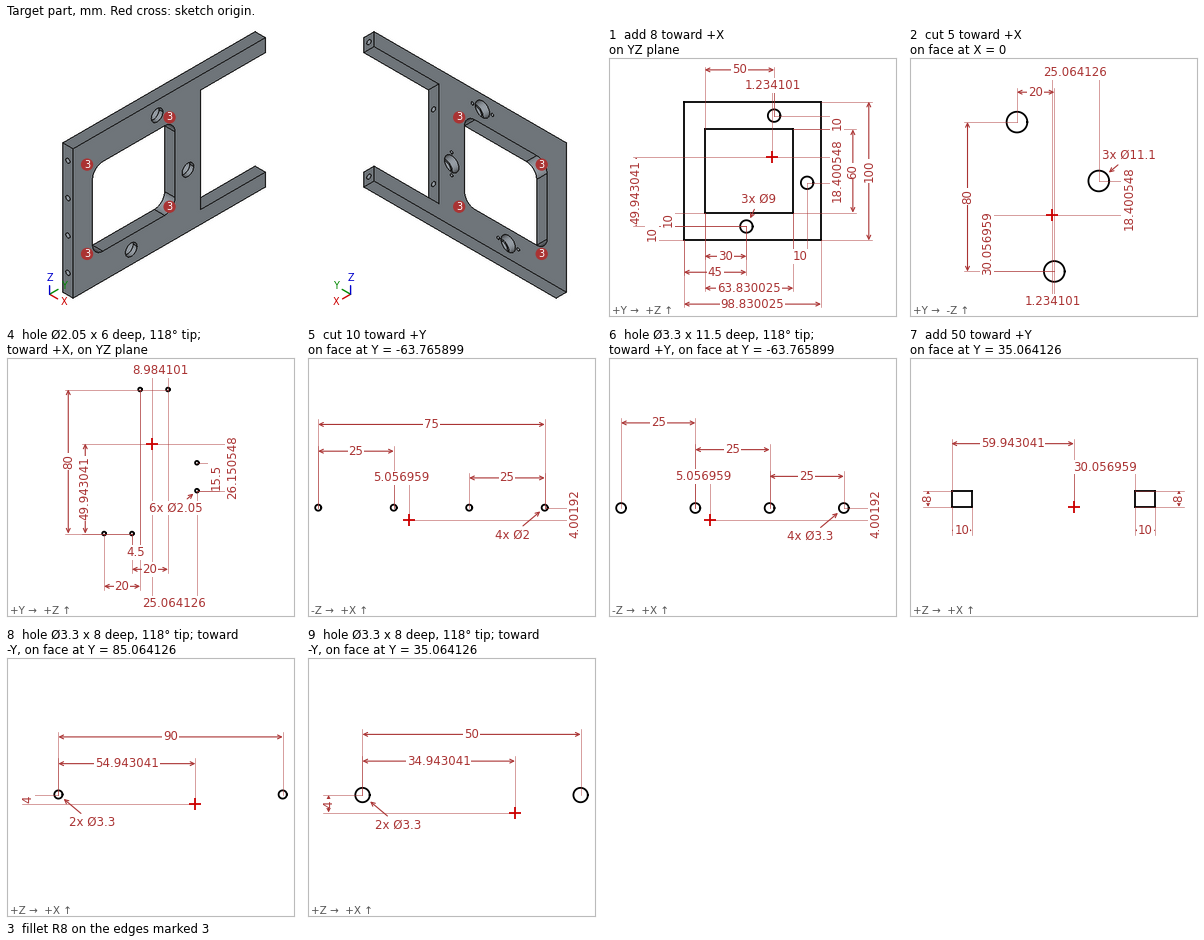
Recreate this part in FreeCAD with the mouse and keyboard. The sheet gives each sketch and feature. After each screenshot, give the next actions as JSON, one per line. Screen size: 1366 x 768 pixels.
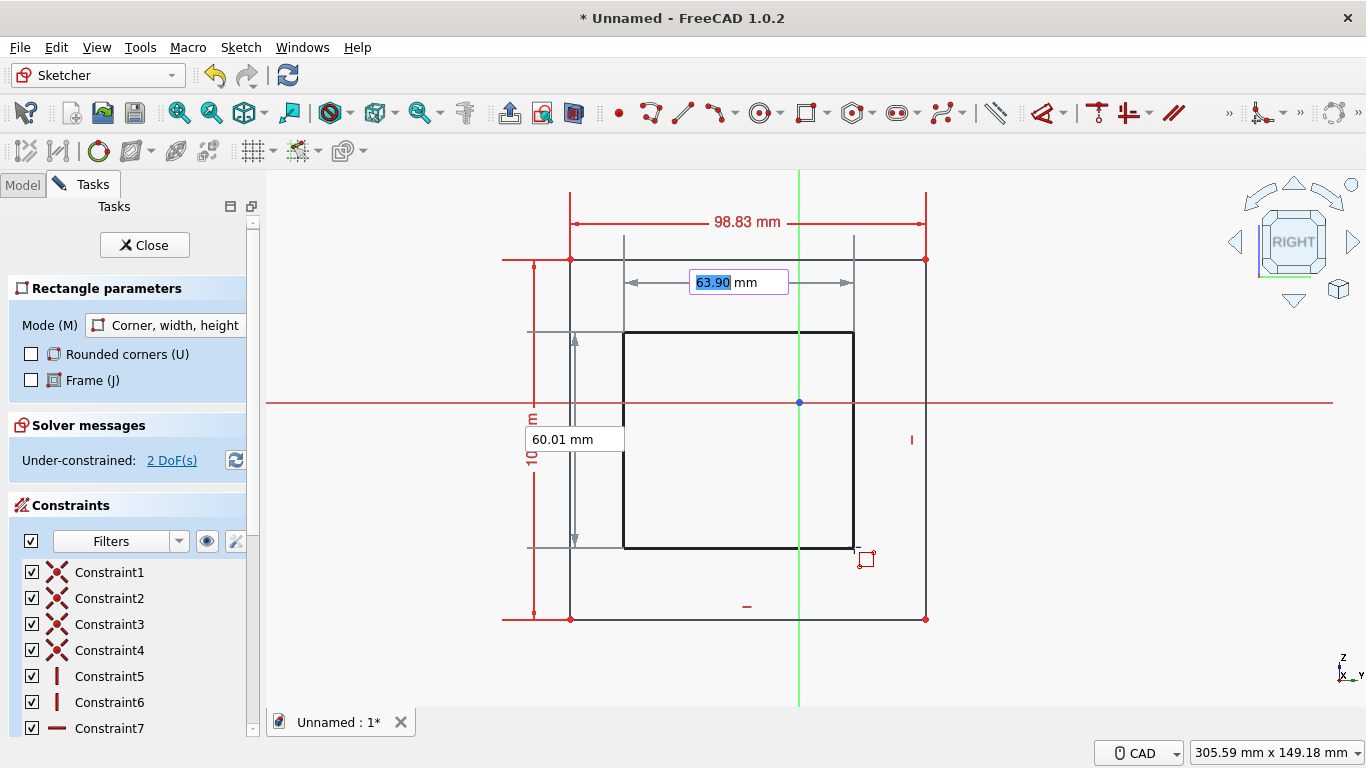
{"action": "type", "text": "63.830025"}
{"action": "key", "text": "Tab"}
{"action": "type", "text": "60"}
{"action": "key", "text": "Return"}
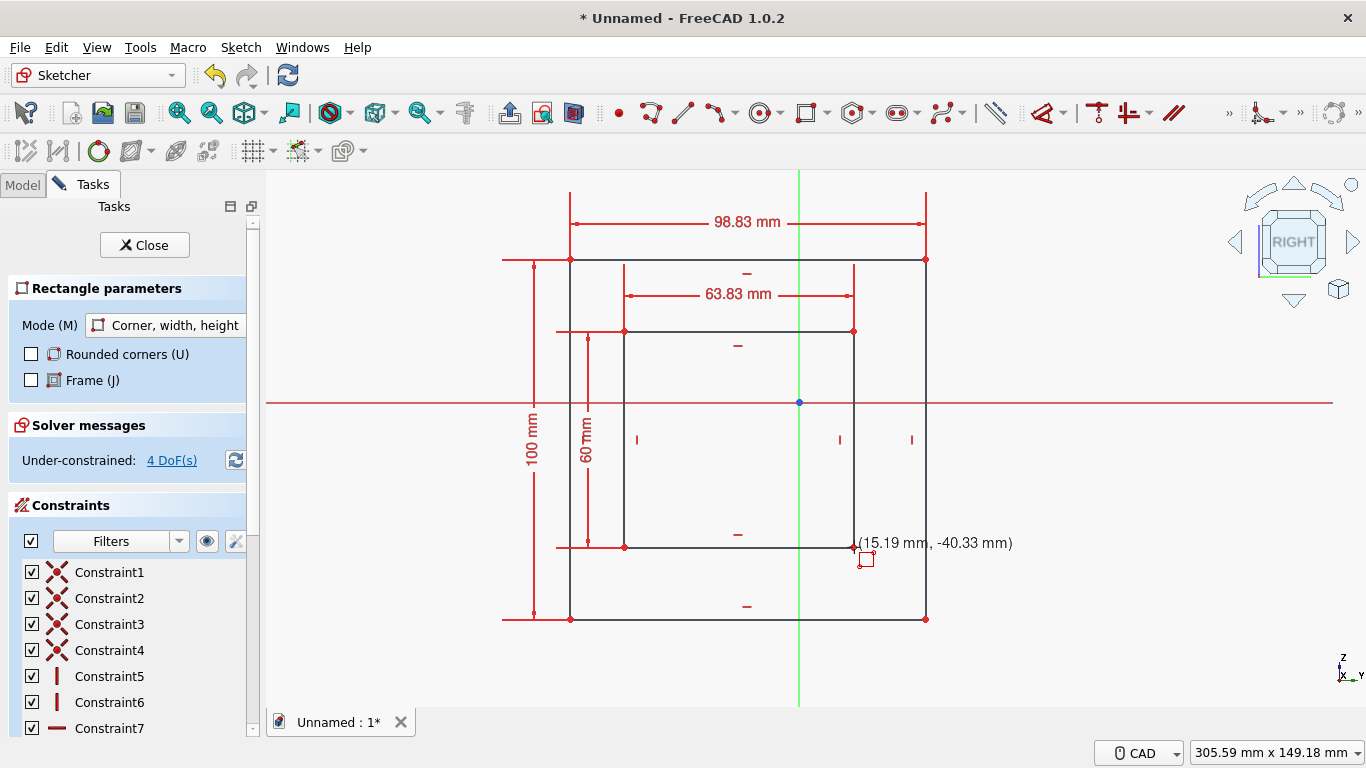
{"action": "left_click", "coordinate": [760, 114]}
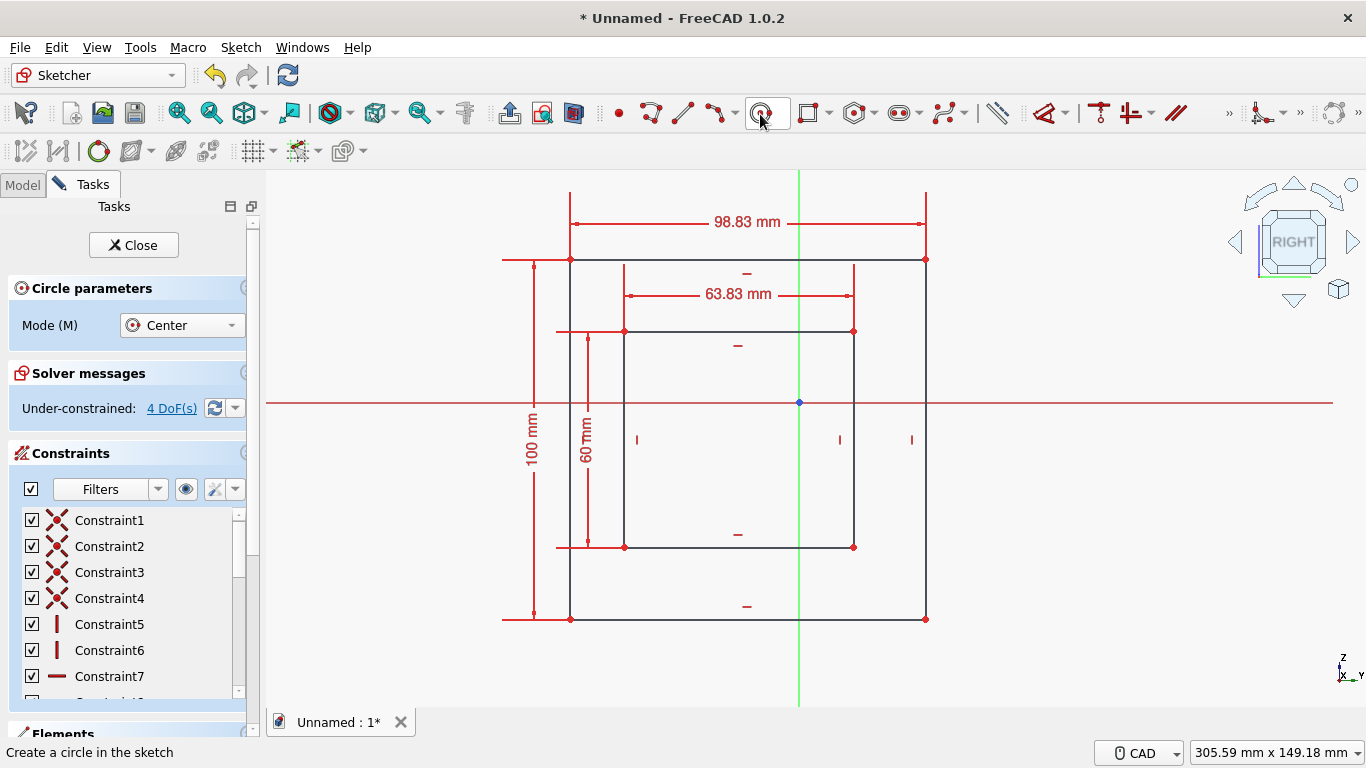
{"action": "scroll", "coordinate": [732, 583], "scroll_direction": "up", "scroll_amount": 2}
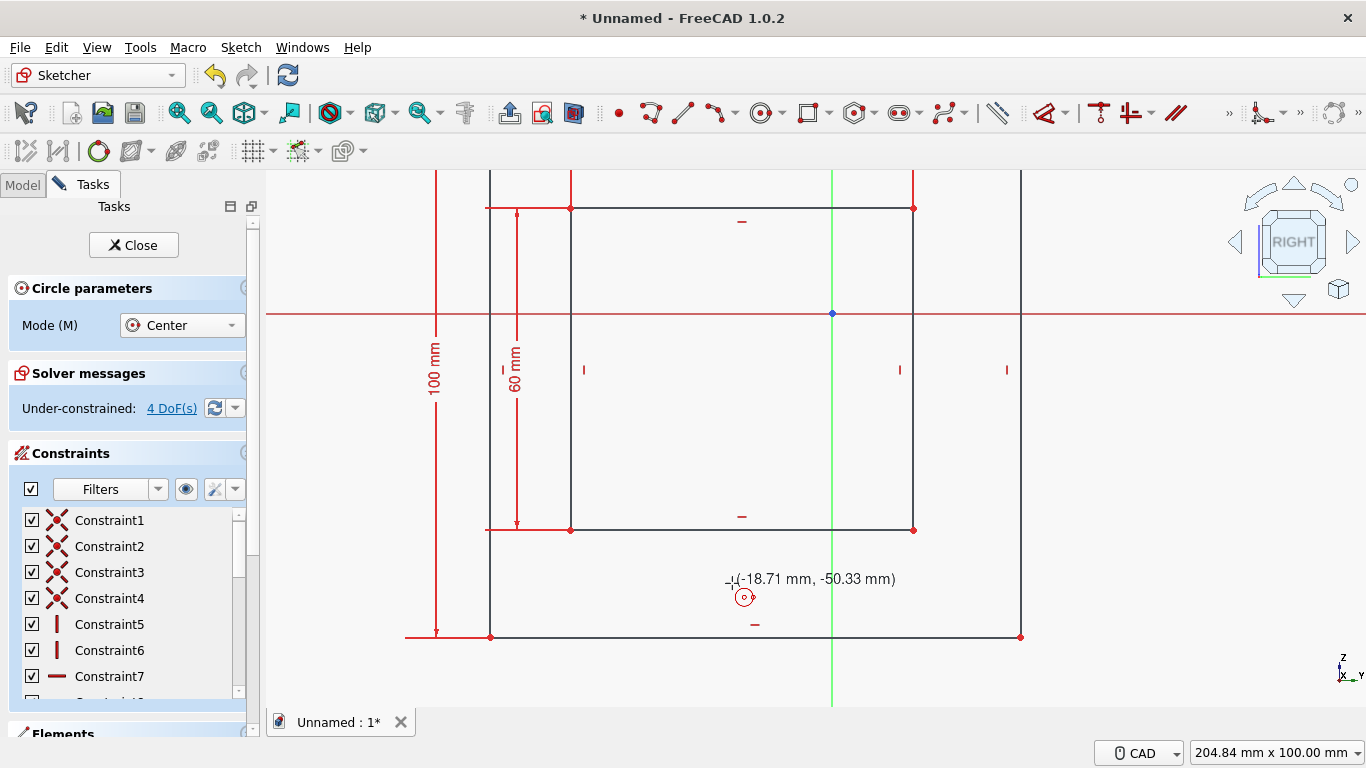
{"action": "left_click", "coordinate": [731, 582]}
{"action": "mouse_move", "coordinate": [749, 565]}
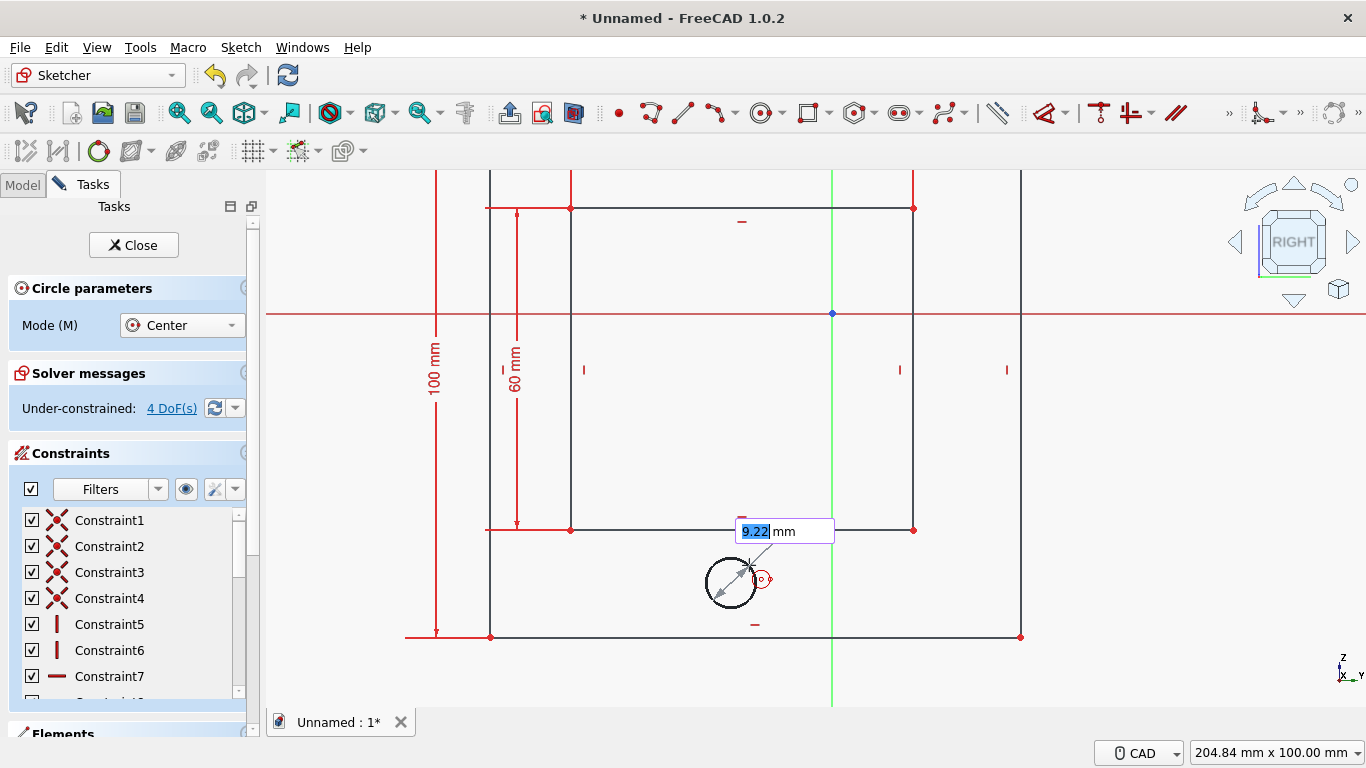
{"action": "type", "text": "9"}
{"action": "key", "text": "Return"}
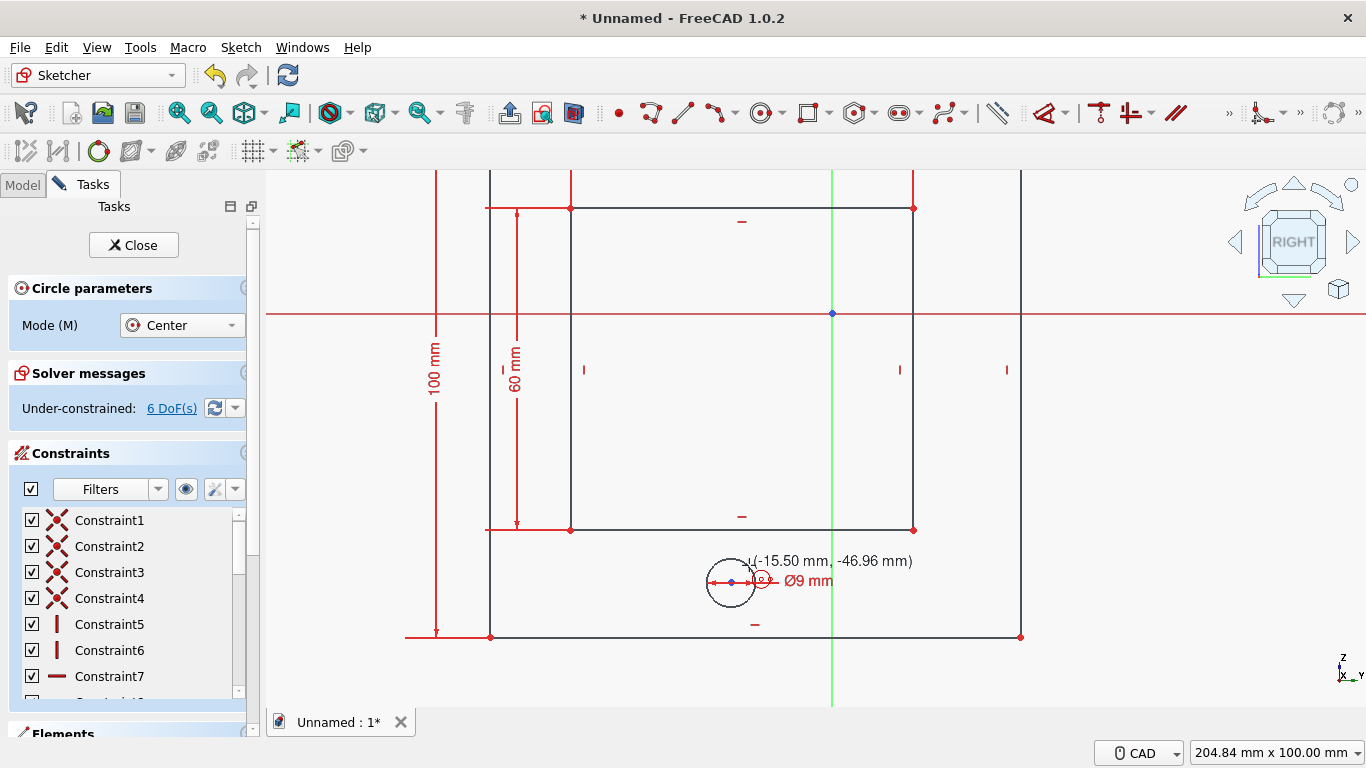
{"action": "scroll", "coordinate": [732, 583], "scroll_direction": "down", "scroll_amount": 2}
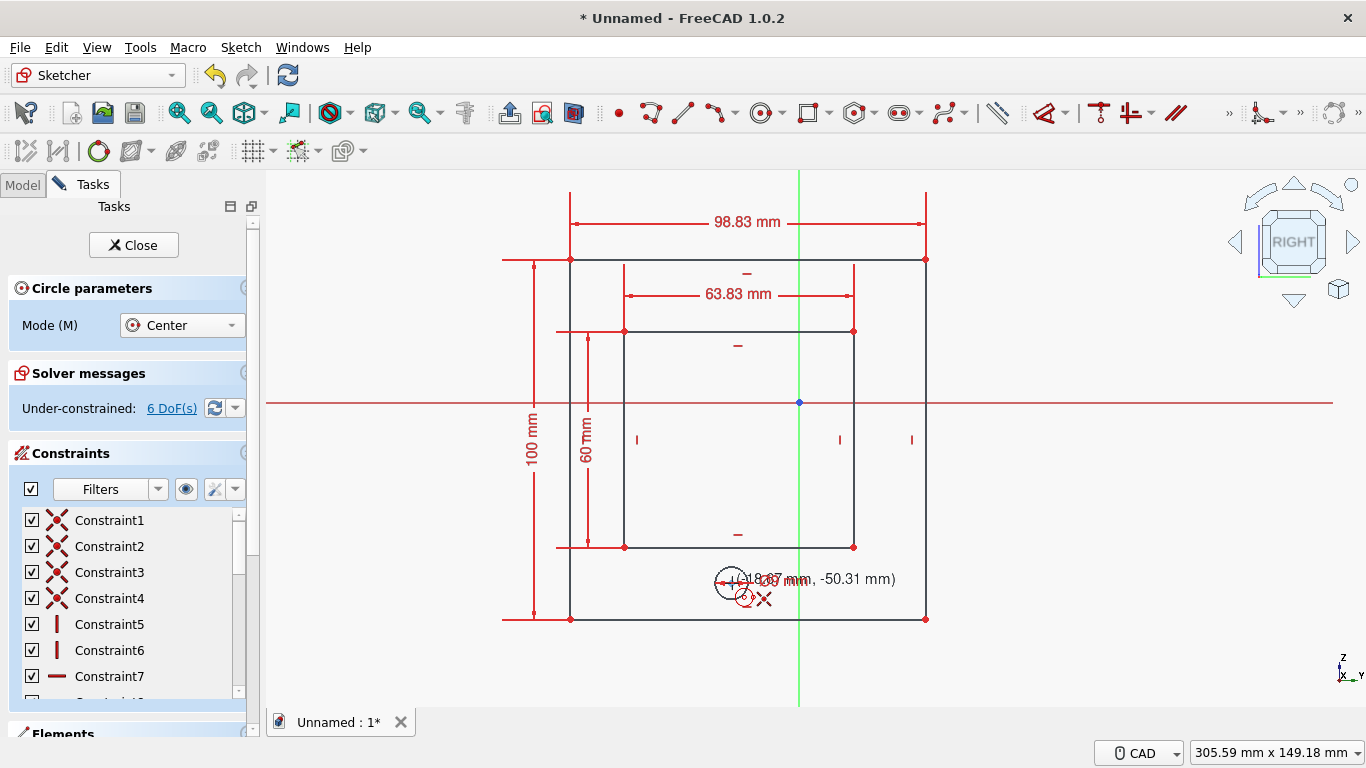
{"action": "scroll", "coordinate": [804, 295], "scroll_direction": "up", "scroll_amount": 7}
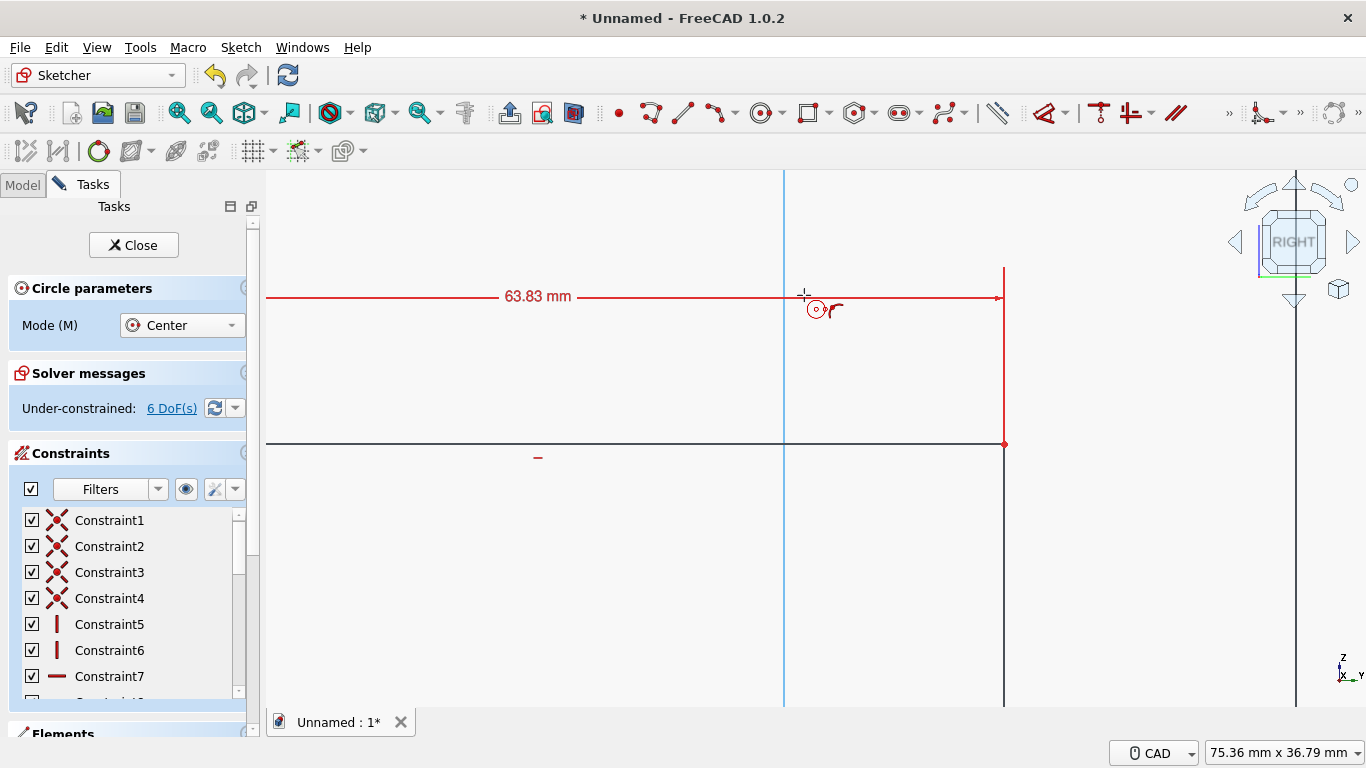
{"action": "left_click", "coordinate": [802, 293]}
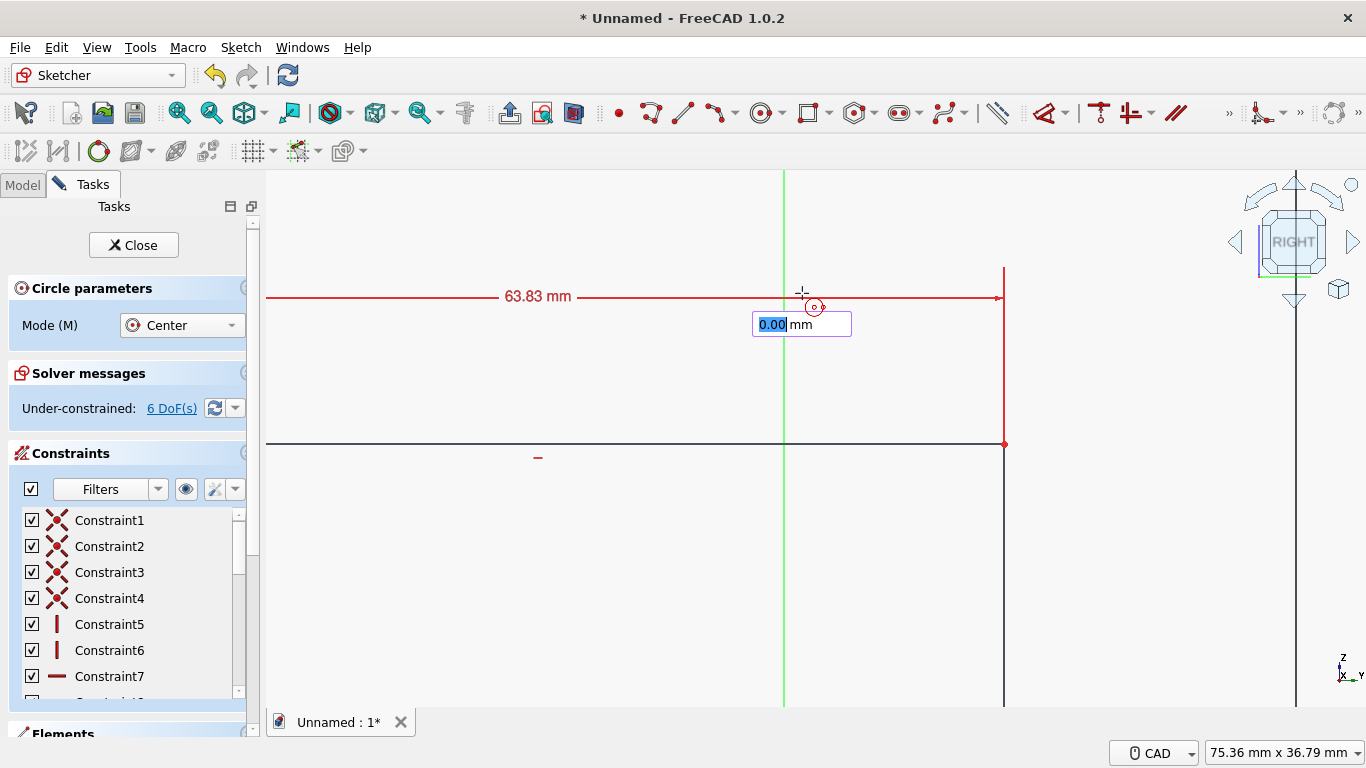
{"action": "scroll", "coordinate": [804, 295], "scroll_direction": "down", "scroll_amount": 7}
{"action": "mouse_move", "coordinate": [815, 283]}